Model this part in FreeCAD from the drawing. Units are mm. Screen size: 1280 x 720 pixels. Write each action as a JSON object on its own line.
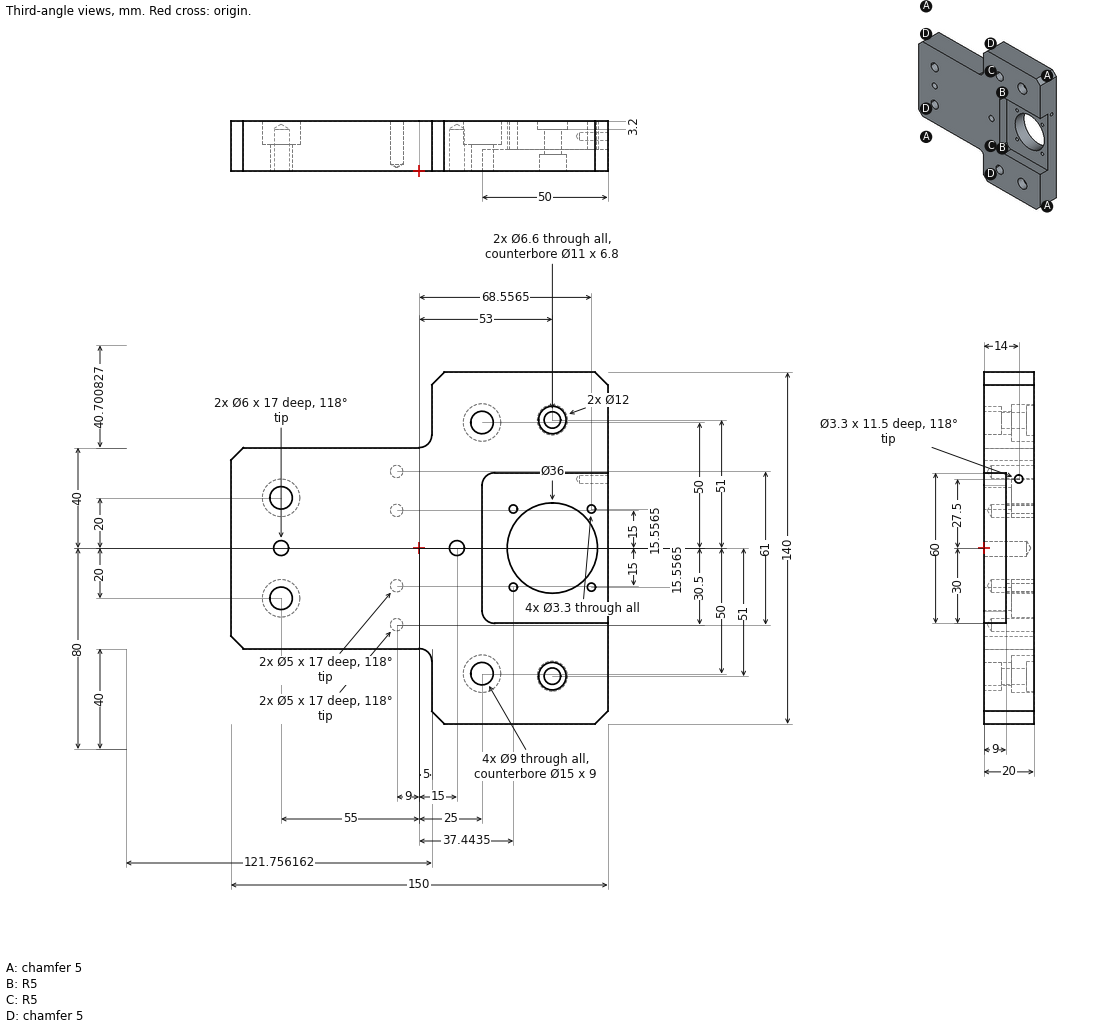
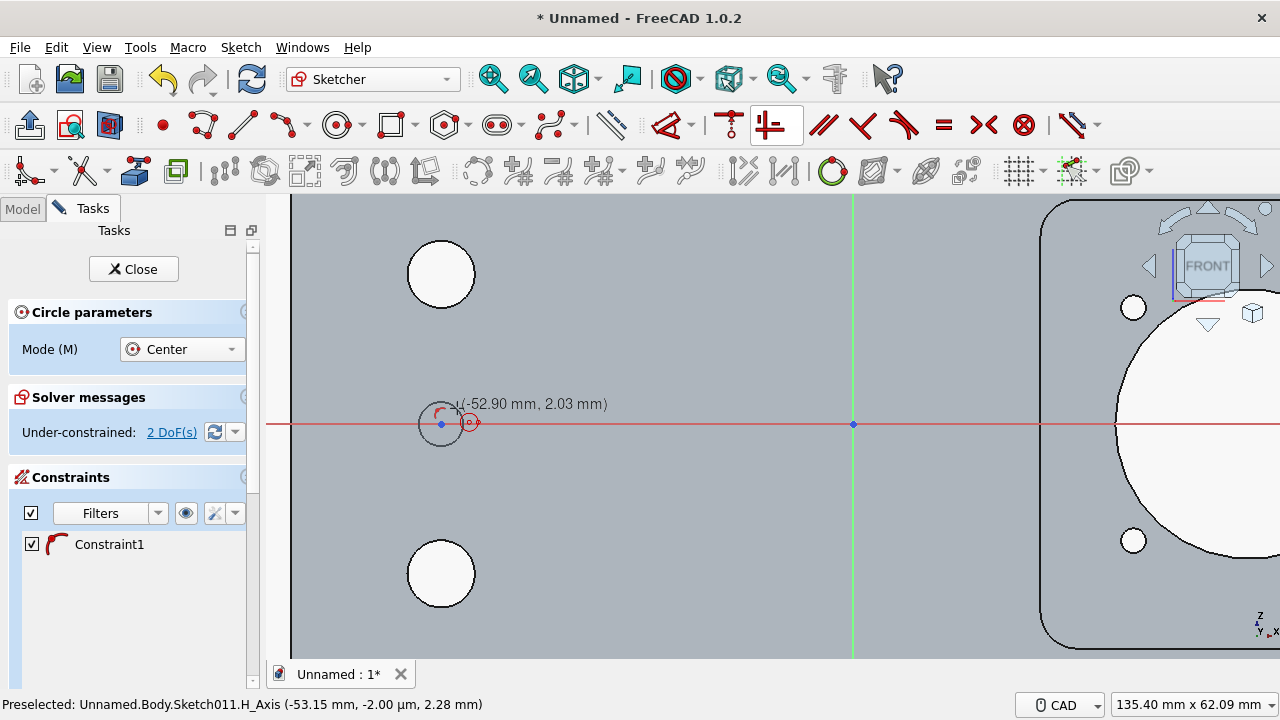
{"action": "left_click", "coordinate": [965, 424]}
{"action": "left_click", "coordinate": [981, 408]}
{"action": "key", "text": "Escape"}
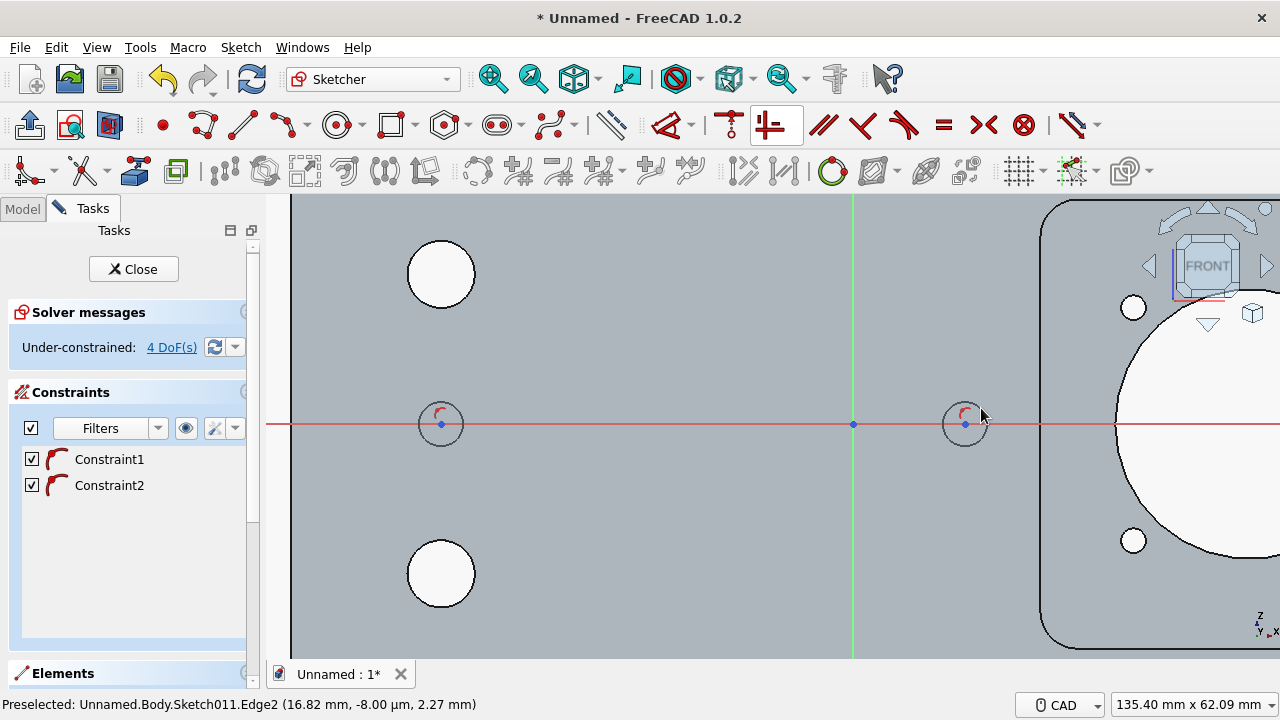
{"action": "left_click", "coordinate": [457, 409]}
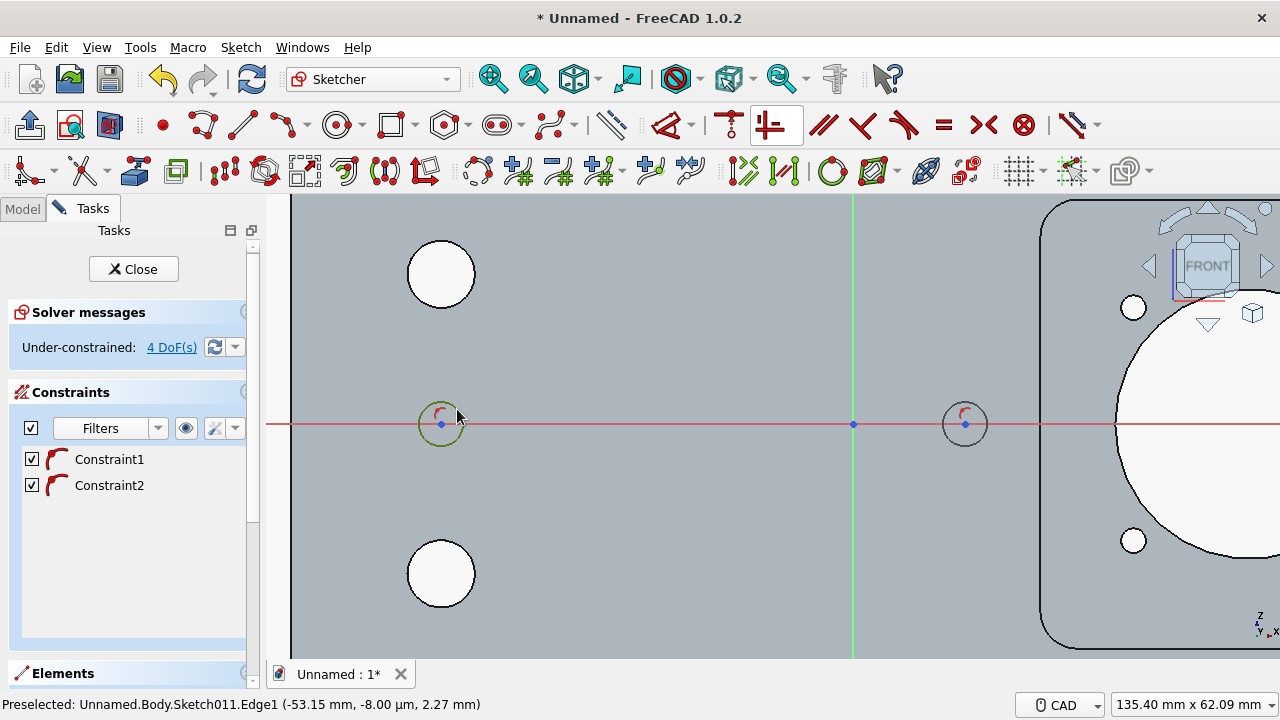
{"action": "left_click", "coordinate": [981, 409]}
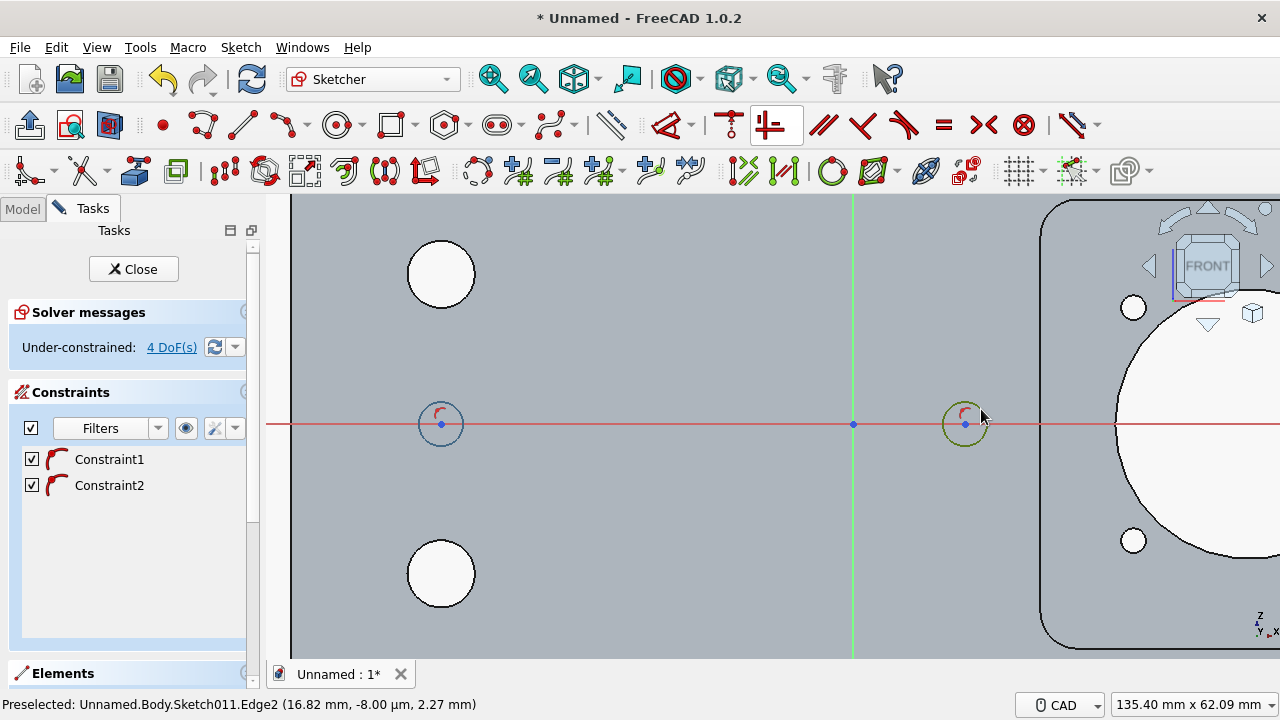
{"action": "left_click", "coordinate": [944, 126]}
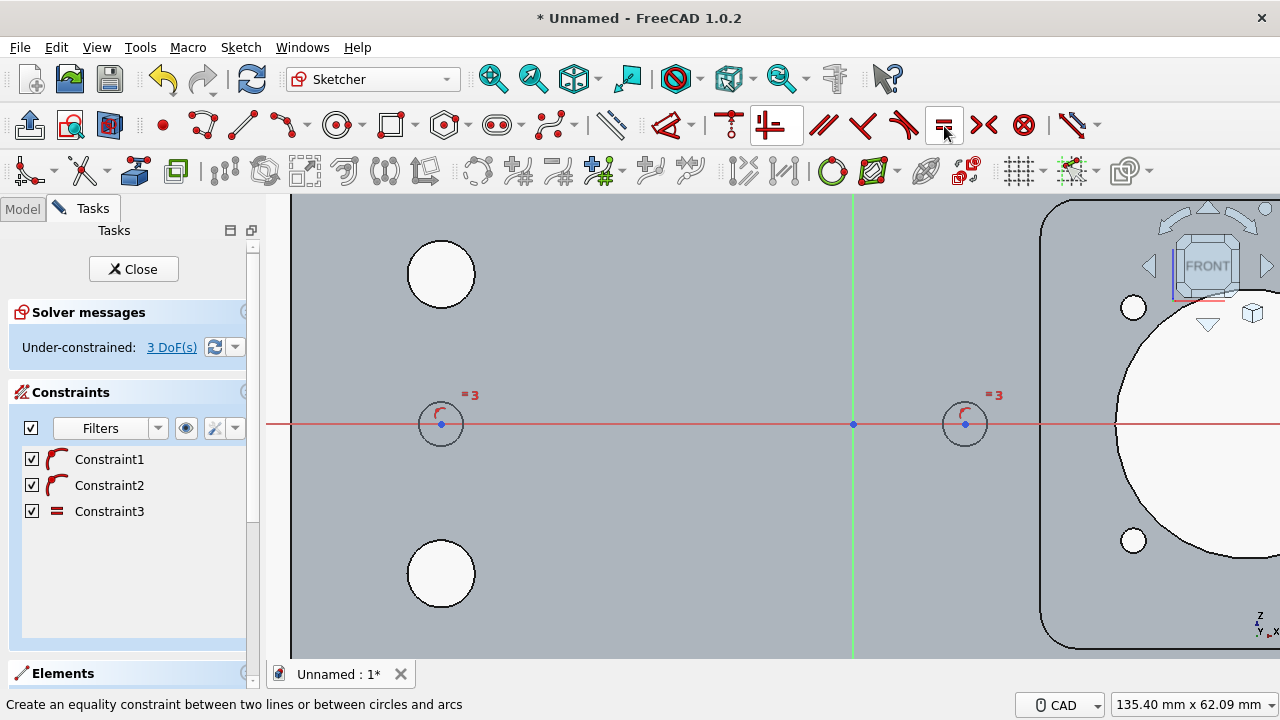
{"action": "left_click", "coordinate": [666, 126]}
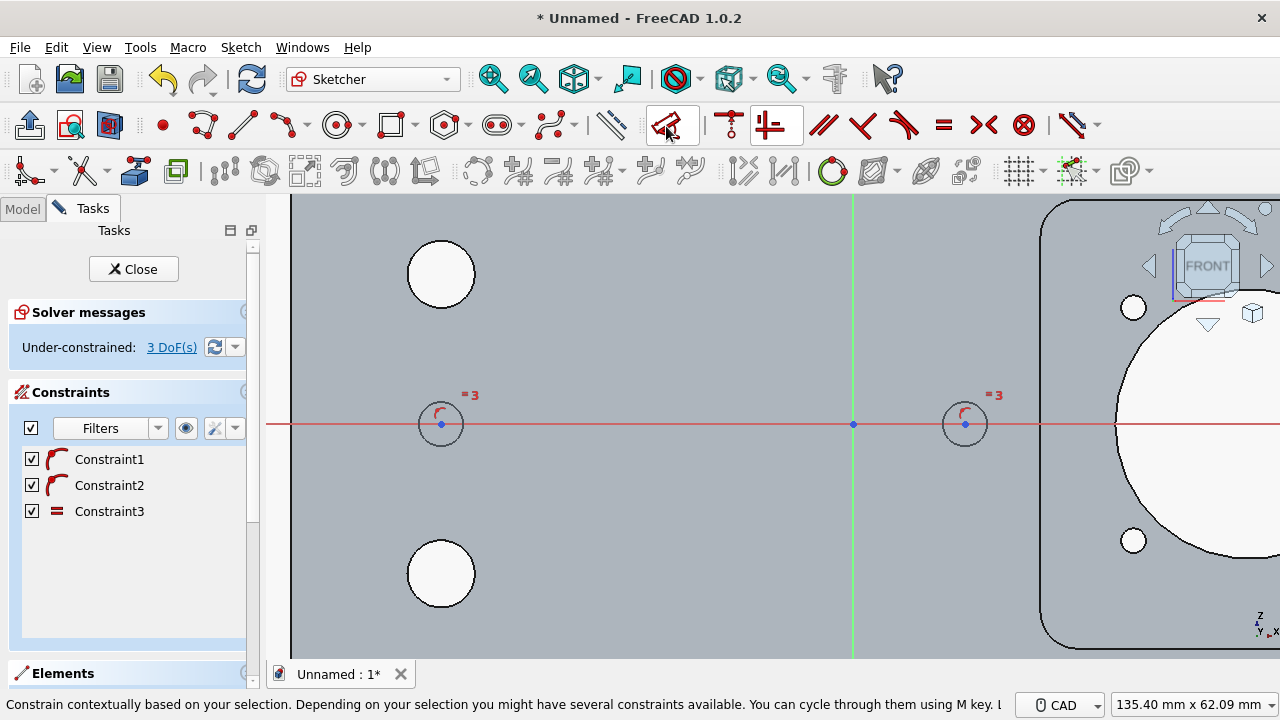
{"action": "left_click", "coordinate": [457, 409]}
{"action": "left_click", "coordinate": [480, 387]}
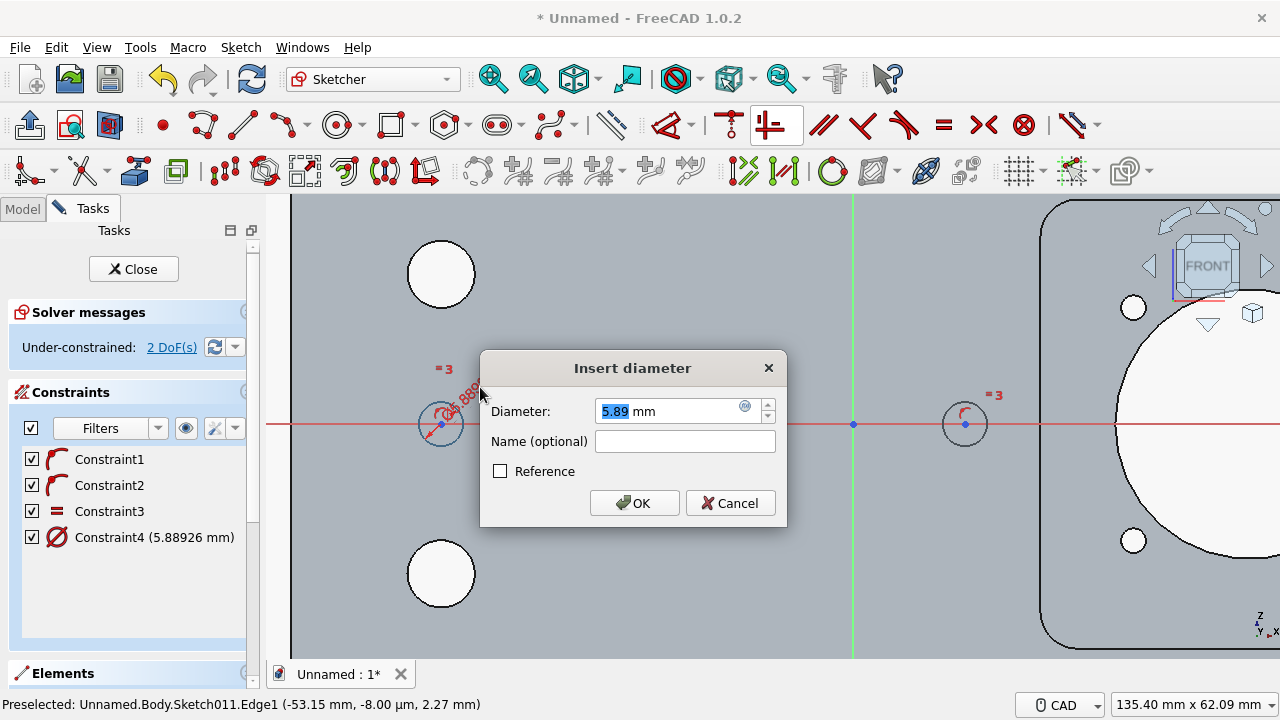
{"action": "type", "text": "6"}
{"action": "key", "text": "Return"}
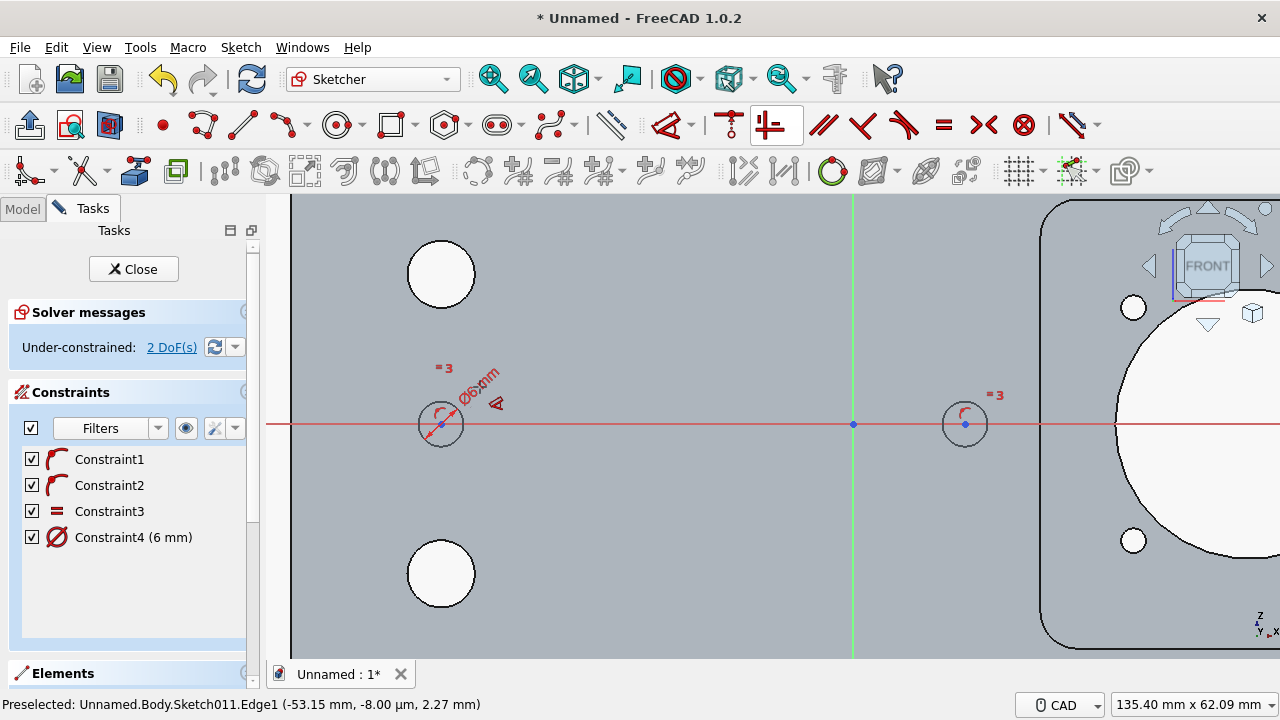
{"action": "left_click", "coordinate": [441, 424]}
{"action": "left_click", "coordinate": [647, 458]}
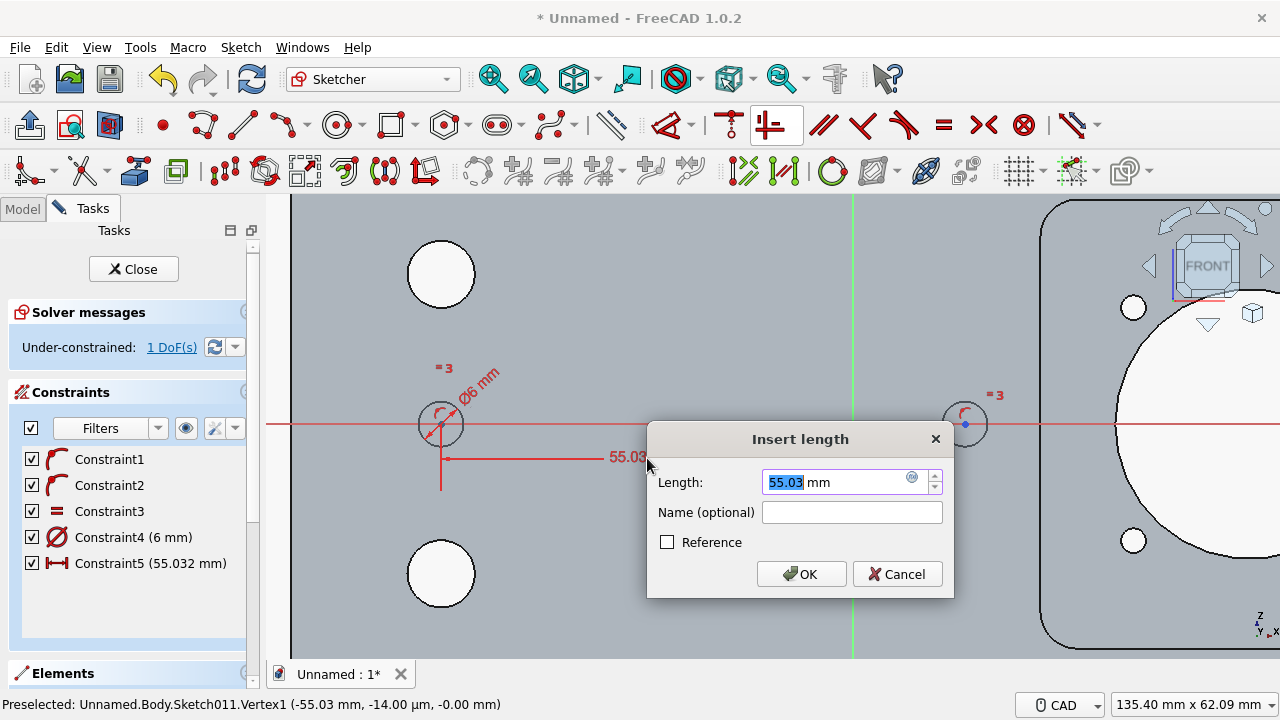
{"action": "type", "text": "55"}
{"action": "key", "text": "Return"}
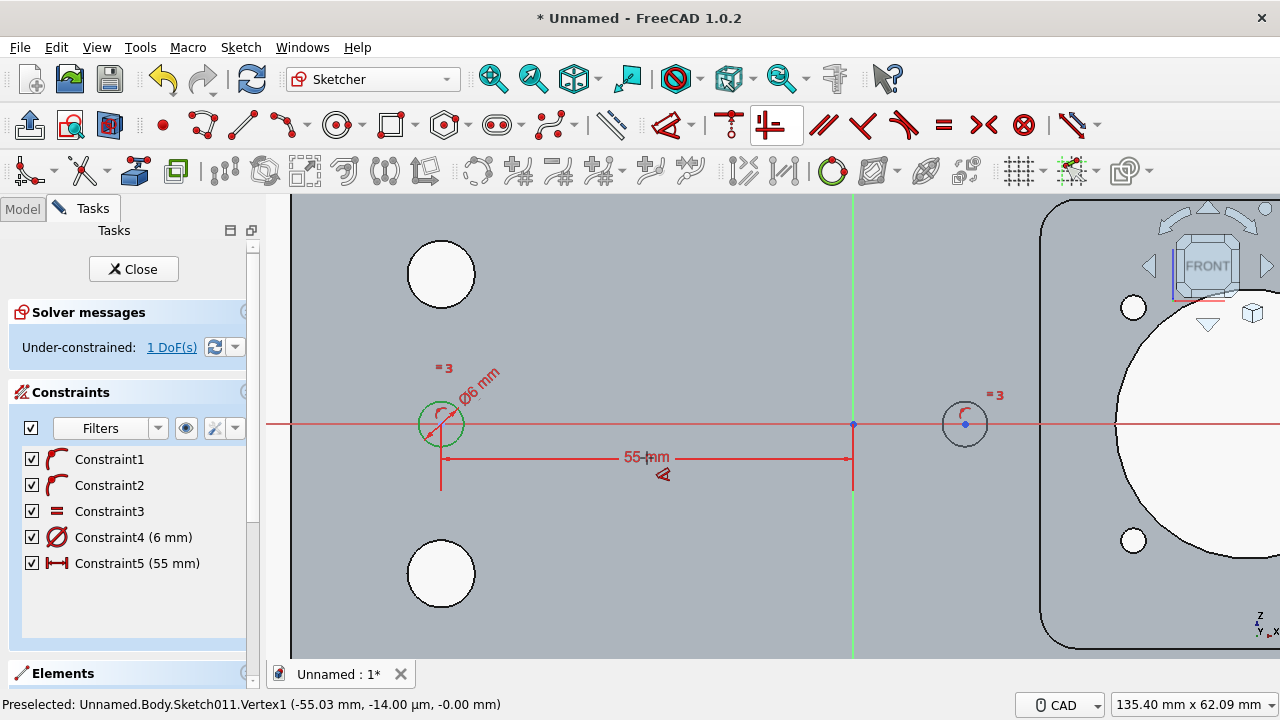
{"action": "left_click", "coordinate": [965, 424]}
{"action": "left_click", "coordinate": [909, 458]}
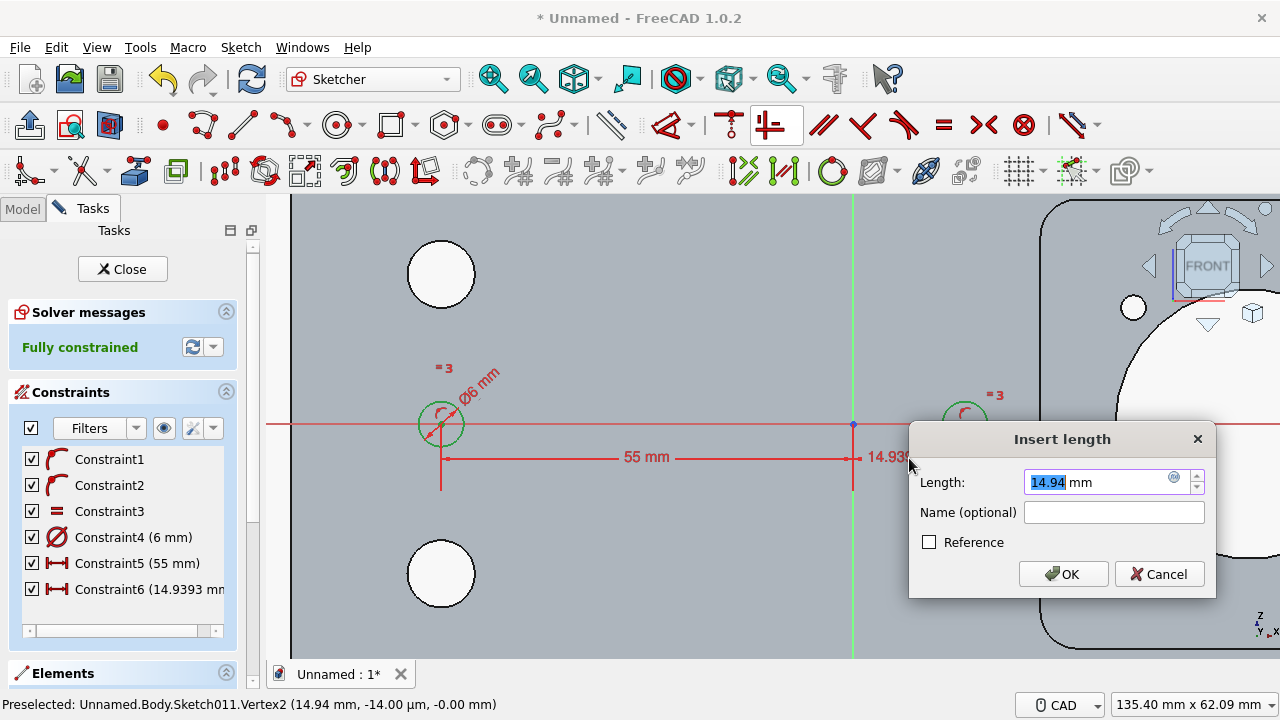
{"action": "type", "text": "15"}
{"action": "key", "text": "Return"}
{"action": "key", "text": "Escape"}